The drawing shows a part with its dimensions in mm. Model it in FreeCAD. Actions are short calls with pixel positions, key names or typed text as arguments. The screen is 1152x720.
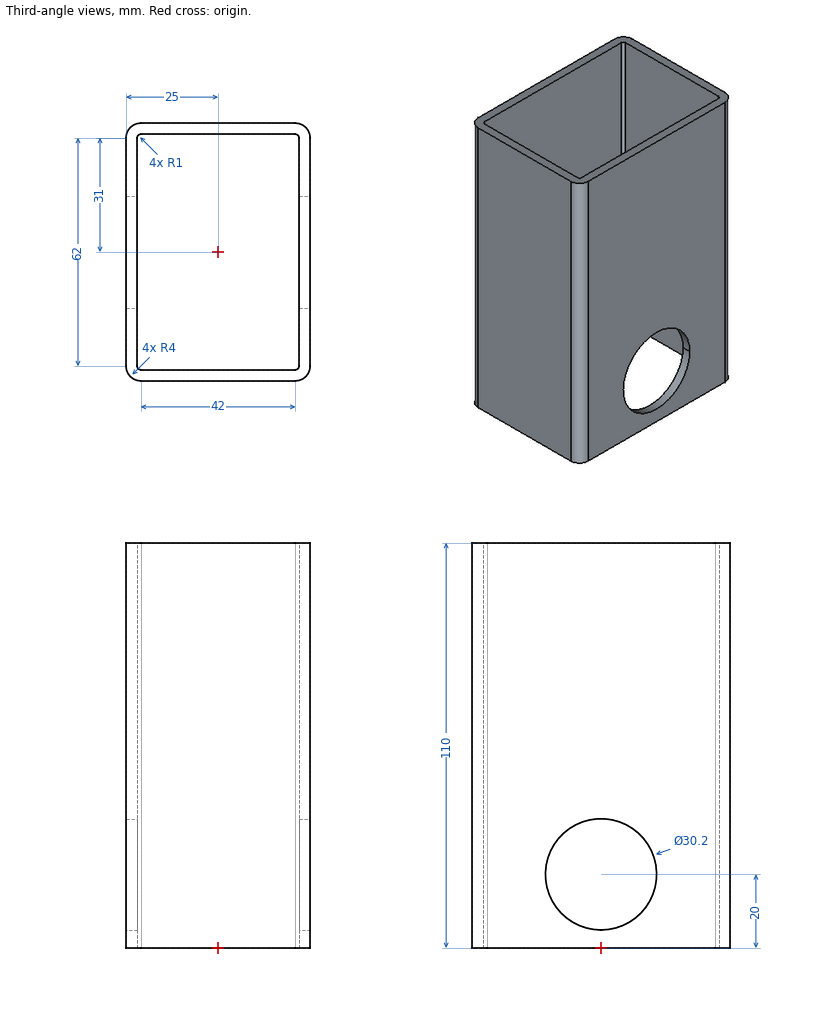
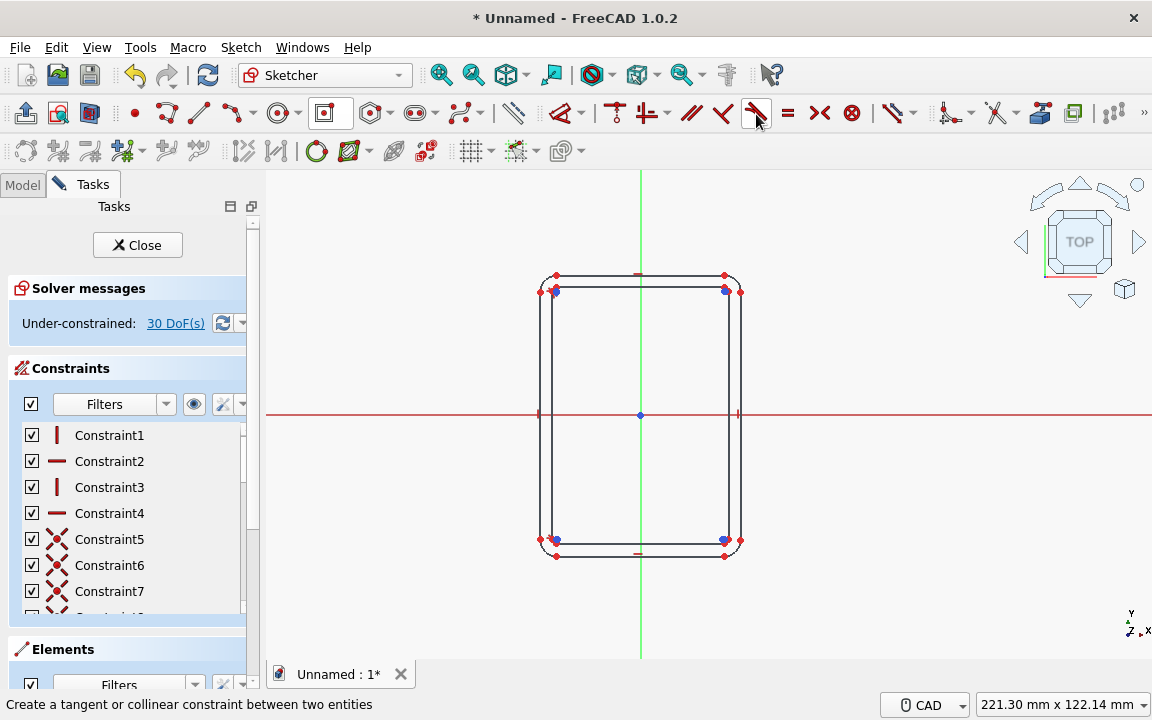
click(607, 557)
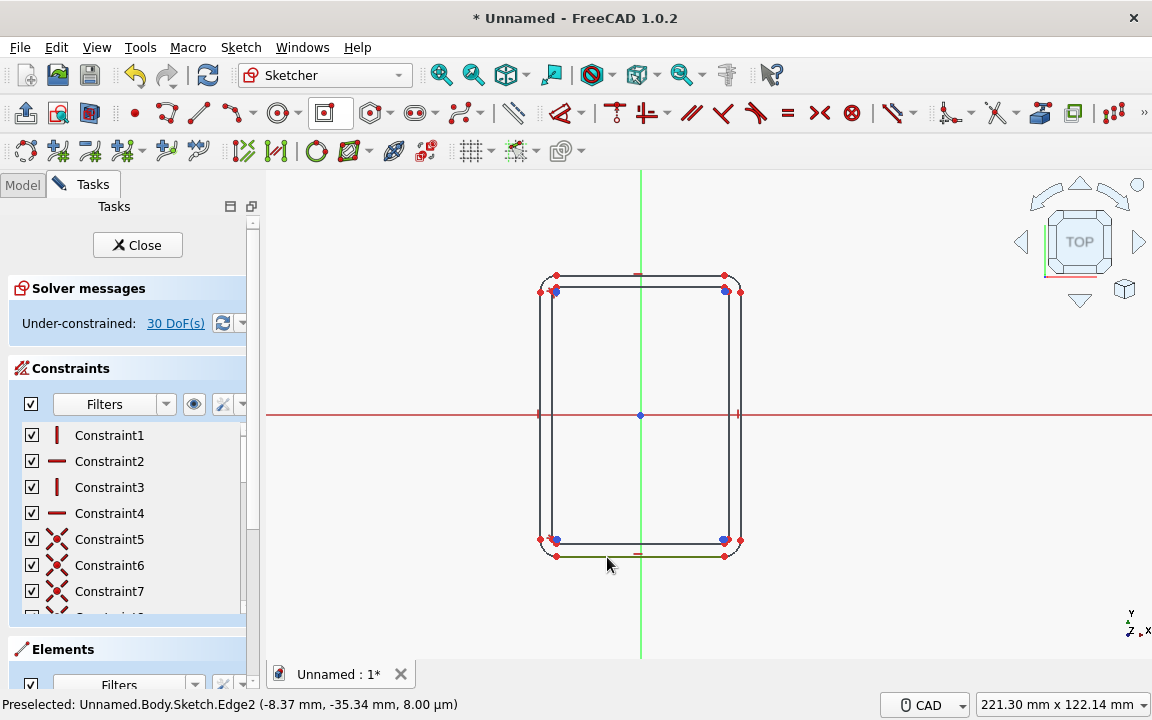
click(545, 551)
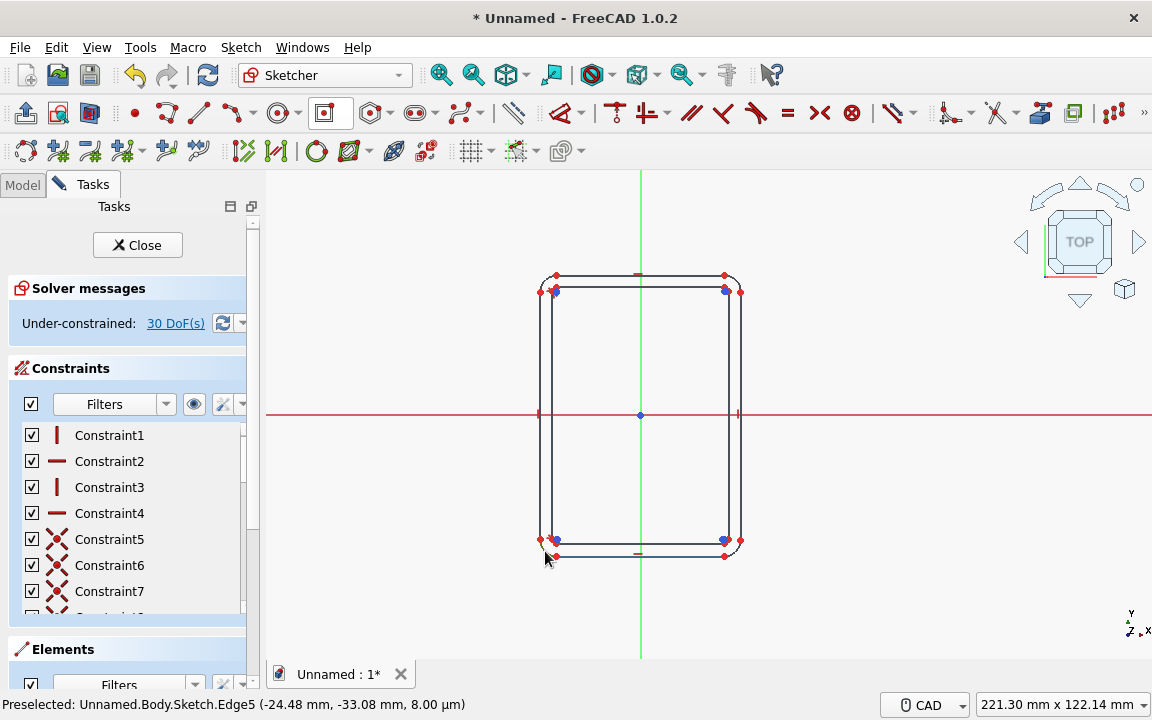
key(t)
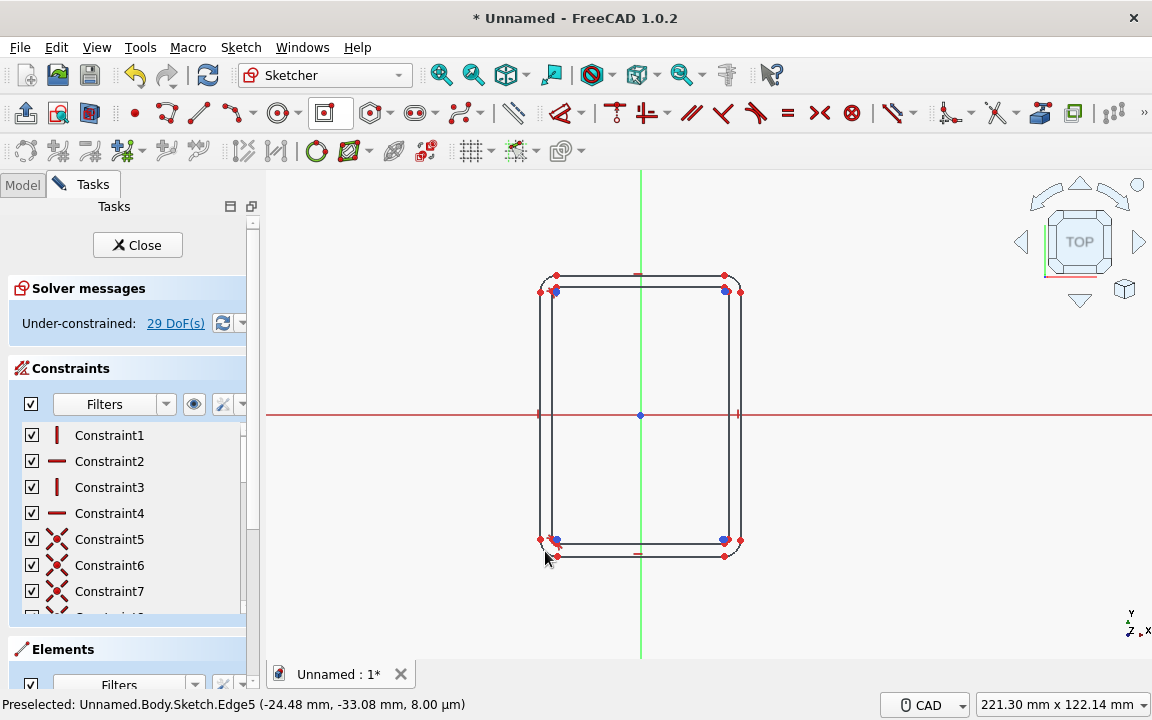
click(608, 557)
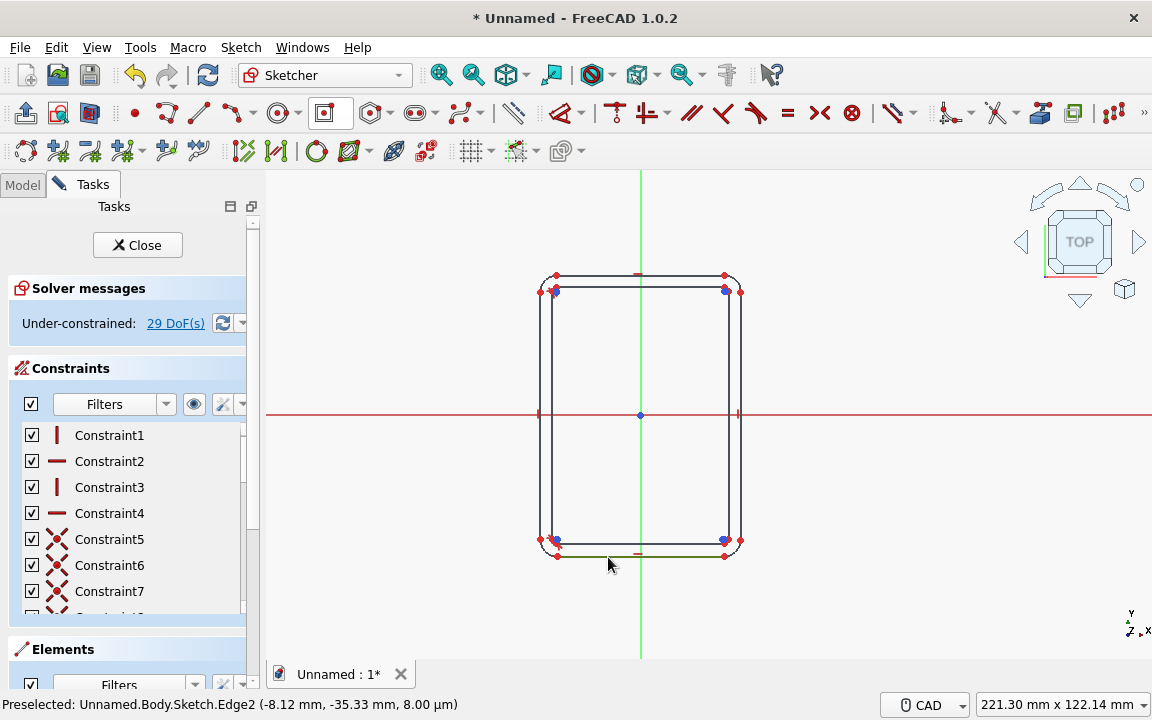
click(736, 551)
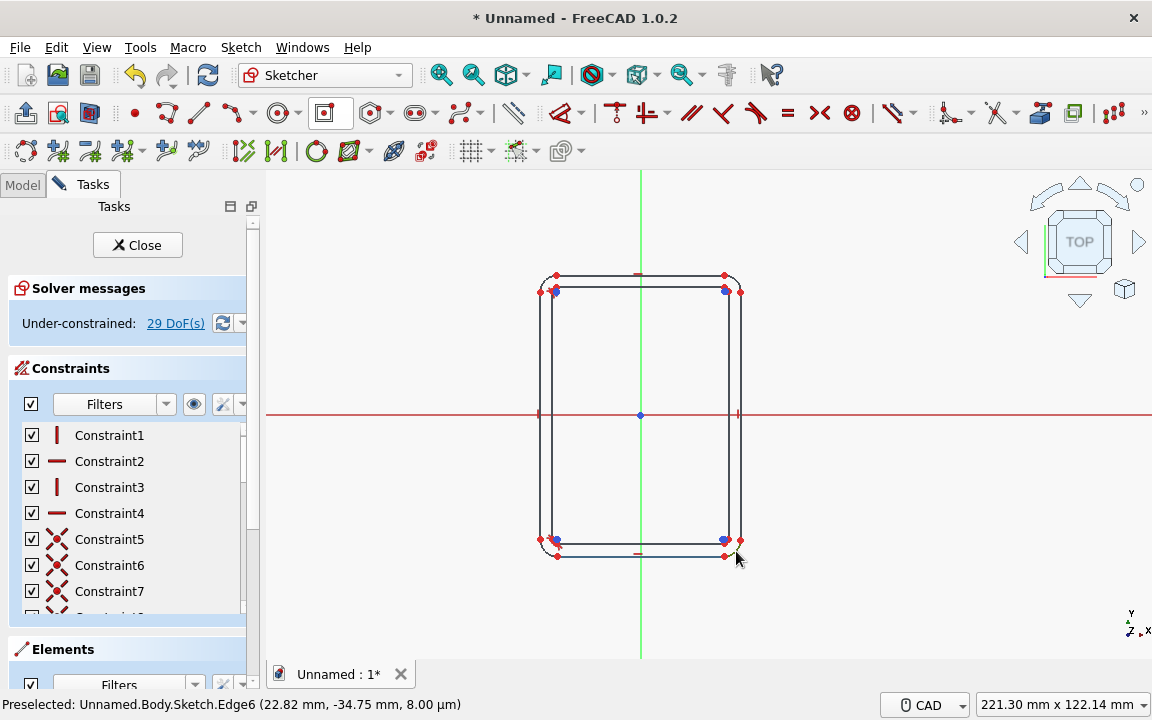
key(t)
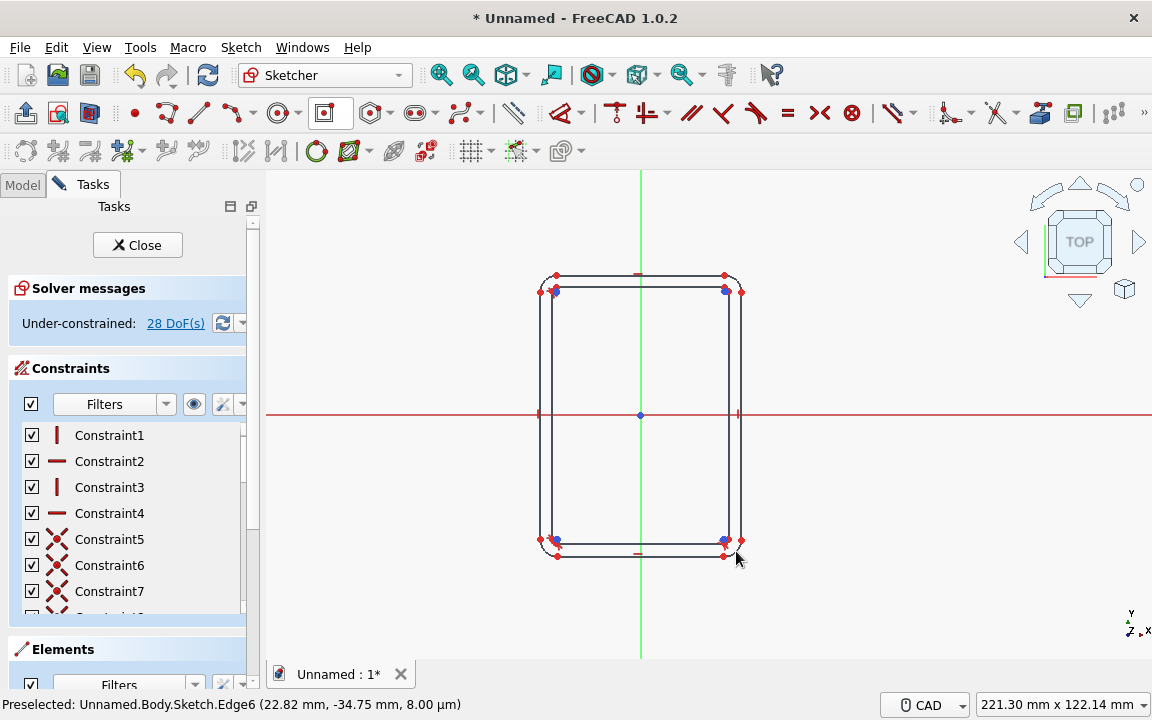
click(741, 466)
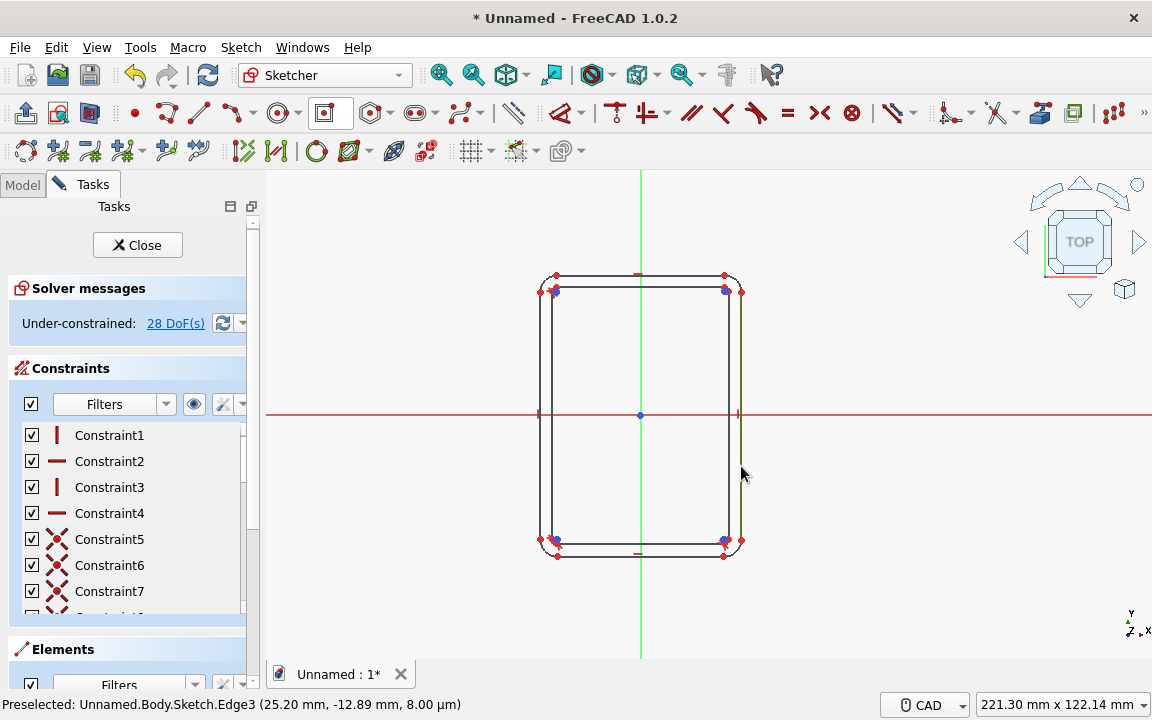
click(736, 552)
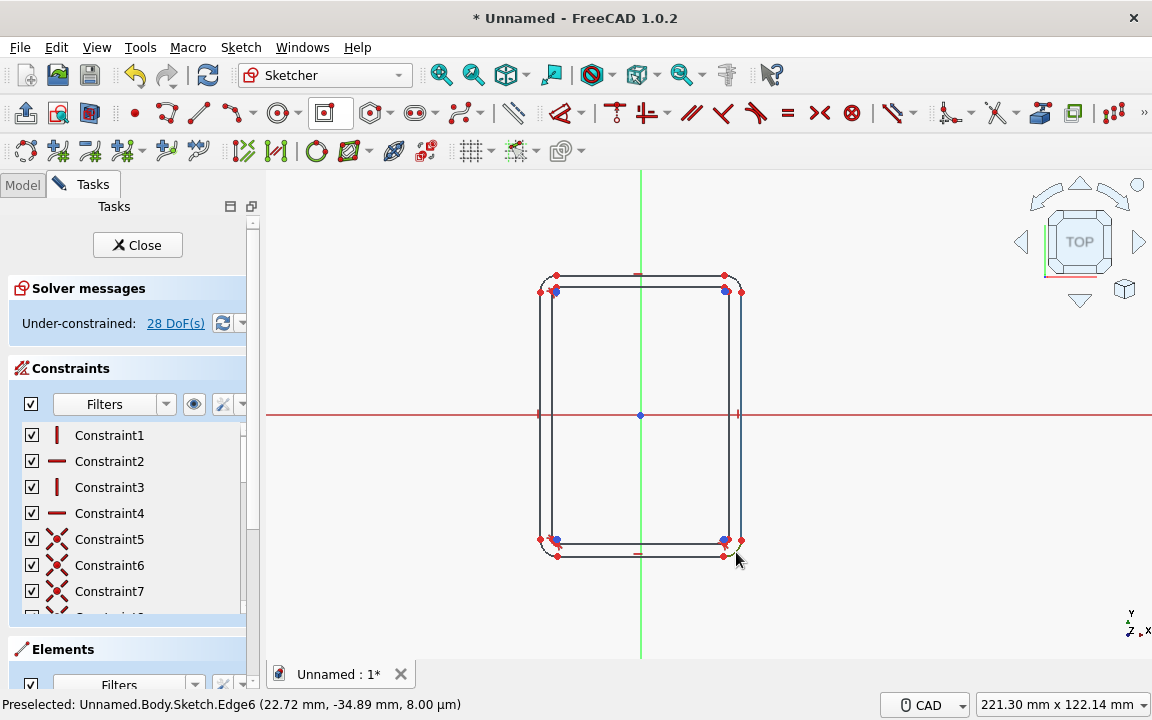
key(t)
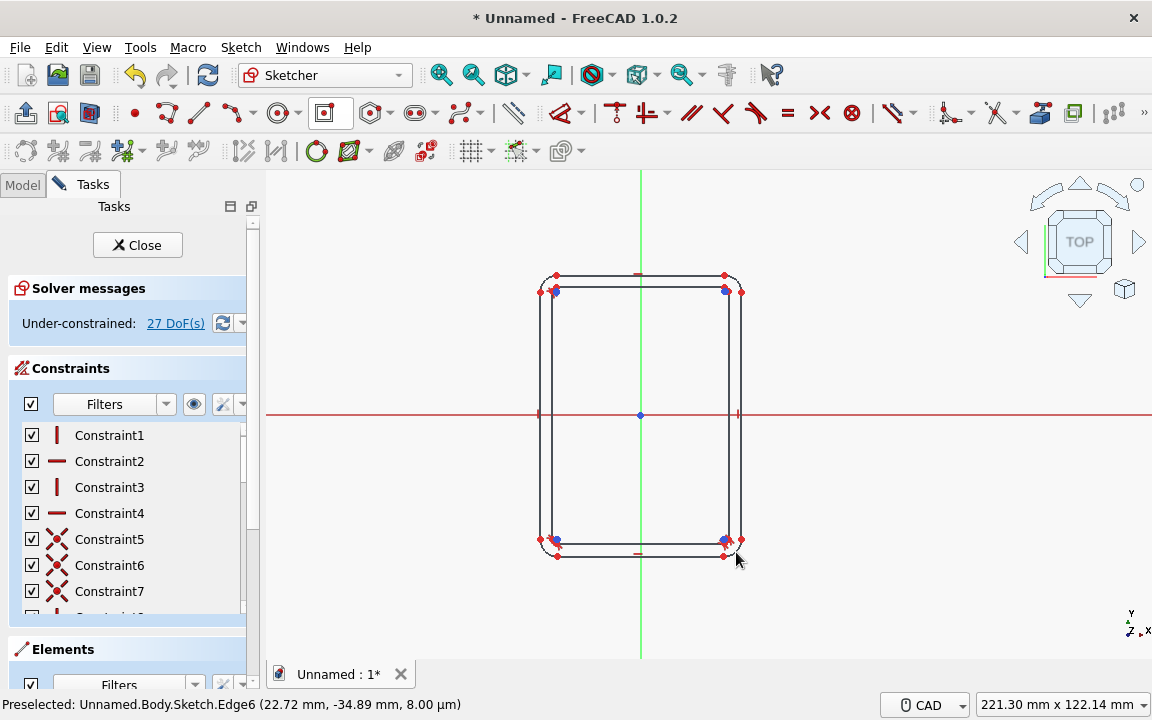
click(741, 465)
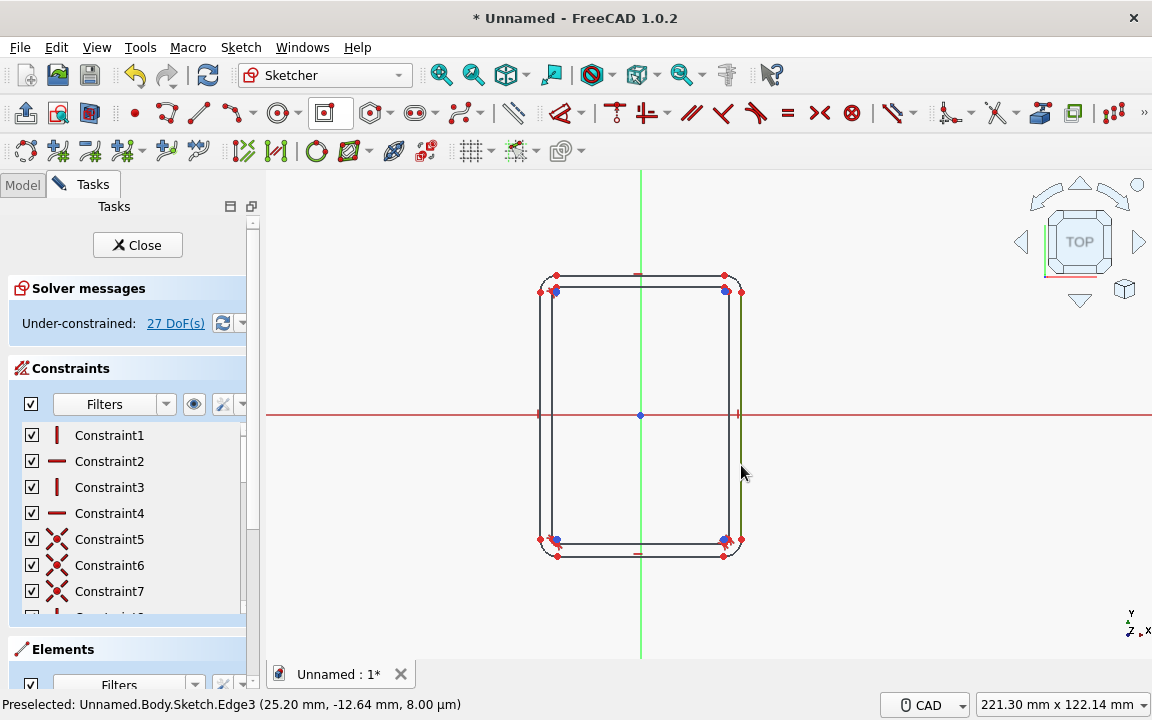
click(737, 280)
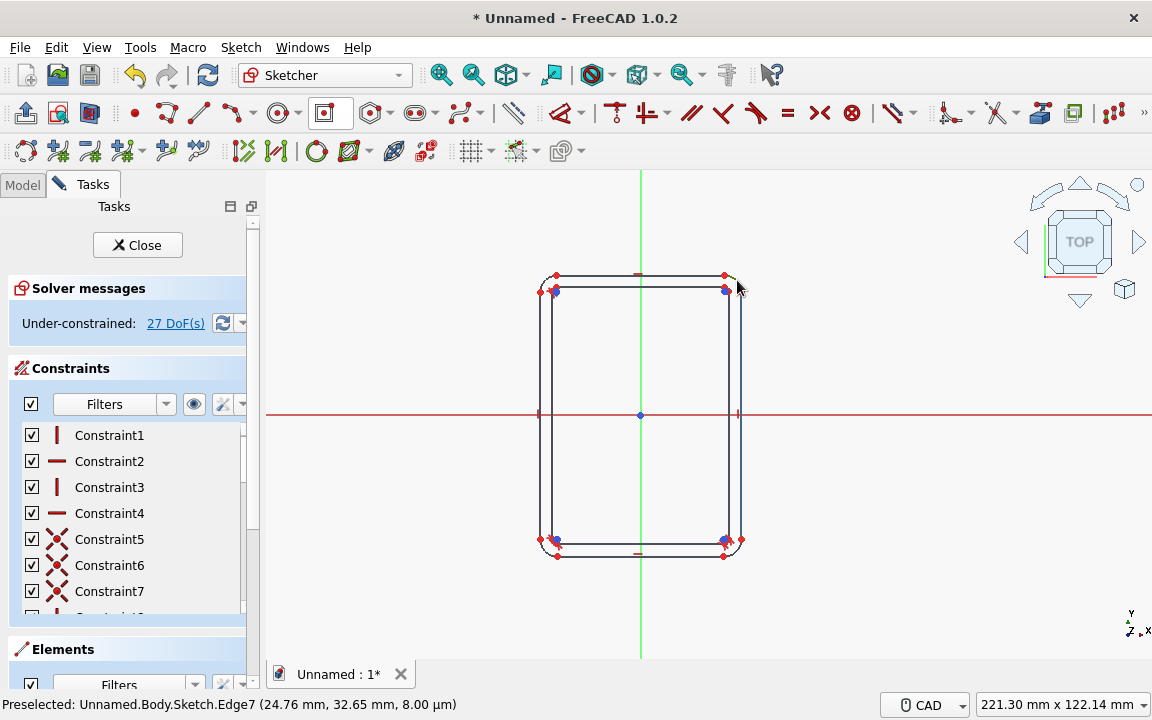
key(t)